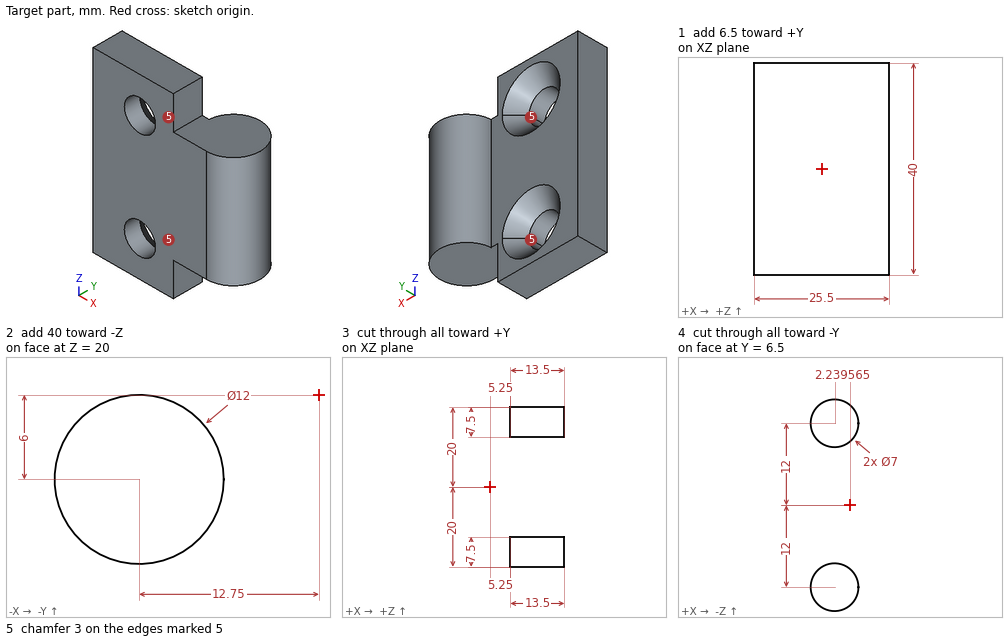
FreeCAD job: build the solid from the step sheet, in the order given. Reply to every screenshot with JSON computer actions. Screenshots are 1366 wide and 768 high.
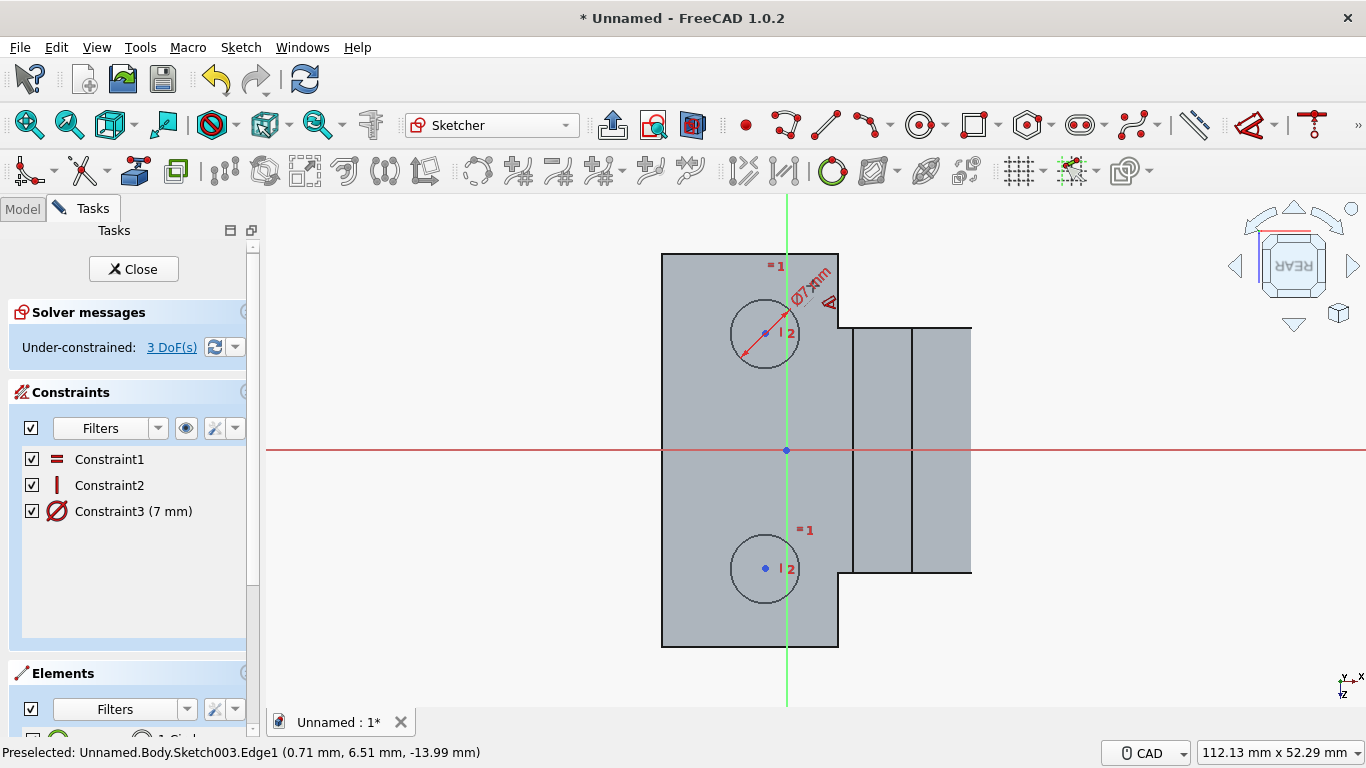
{"action": "left_click", "coordinate": [765, 334]}
{"action": "left_click", "coordinate": [821, 392]}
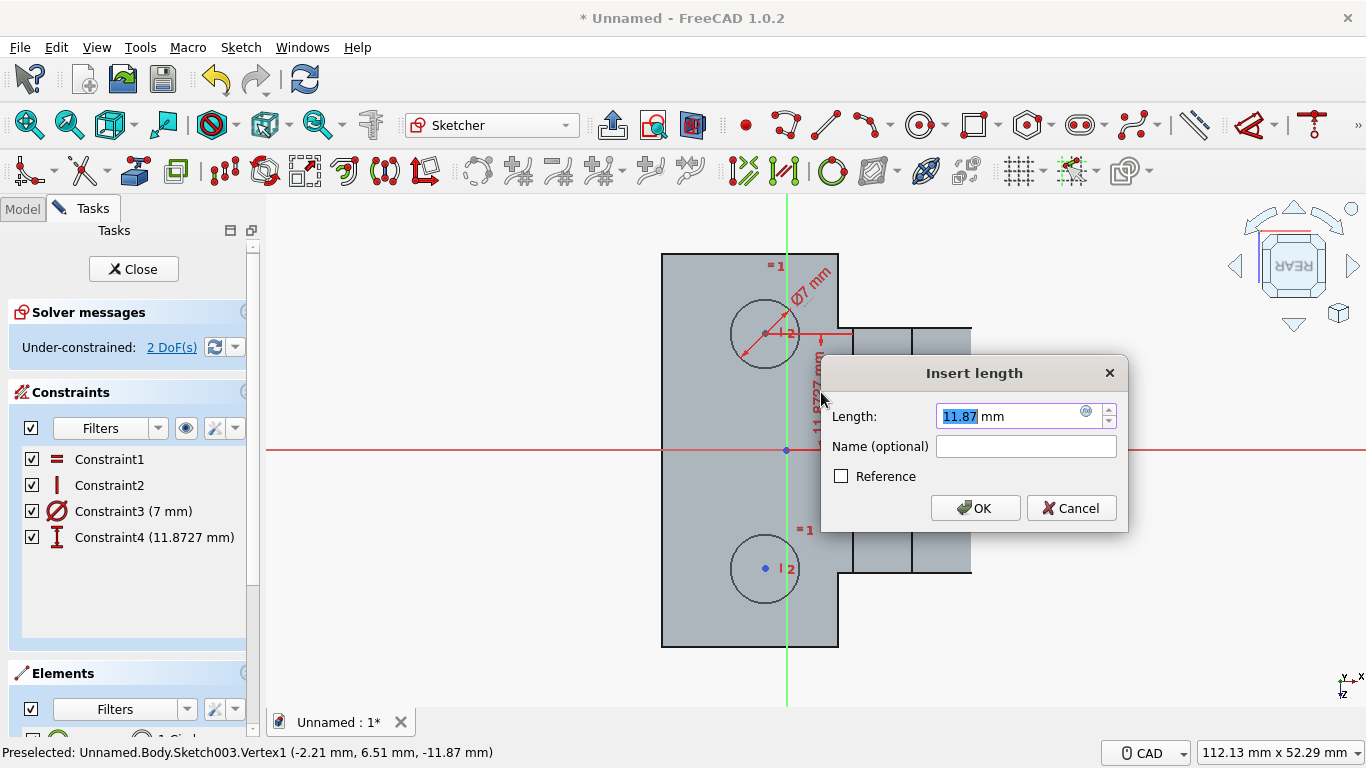
{"action": "type", "text": "12"}
{"action": "key", "text": "Return"}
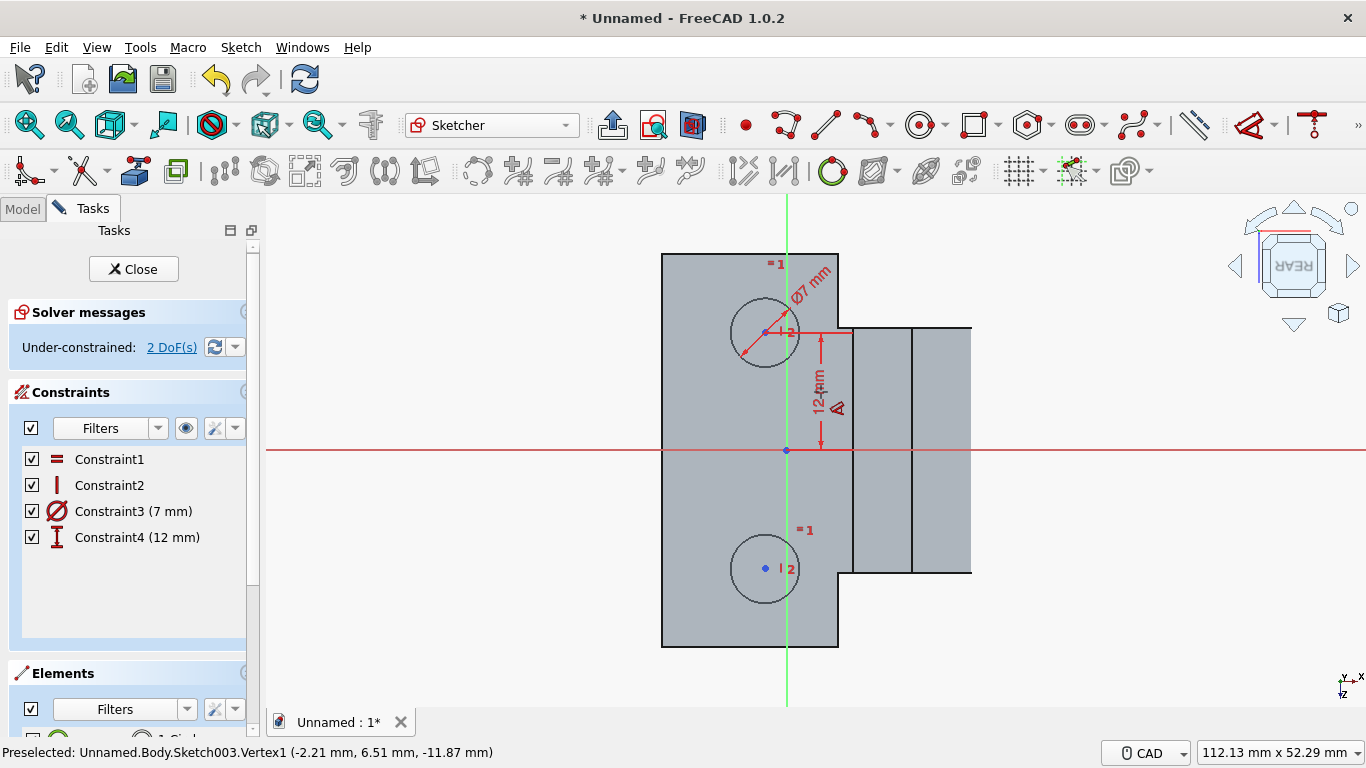
{"action": "left_click", "coordinate": [765, 569]}
{"action": "left_click", "coordinate": [821, 510]}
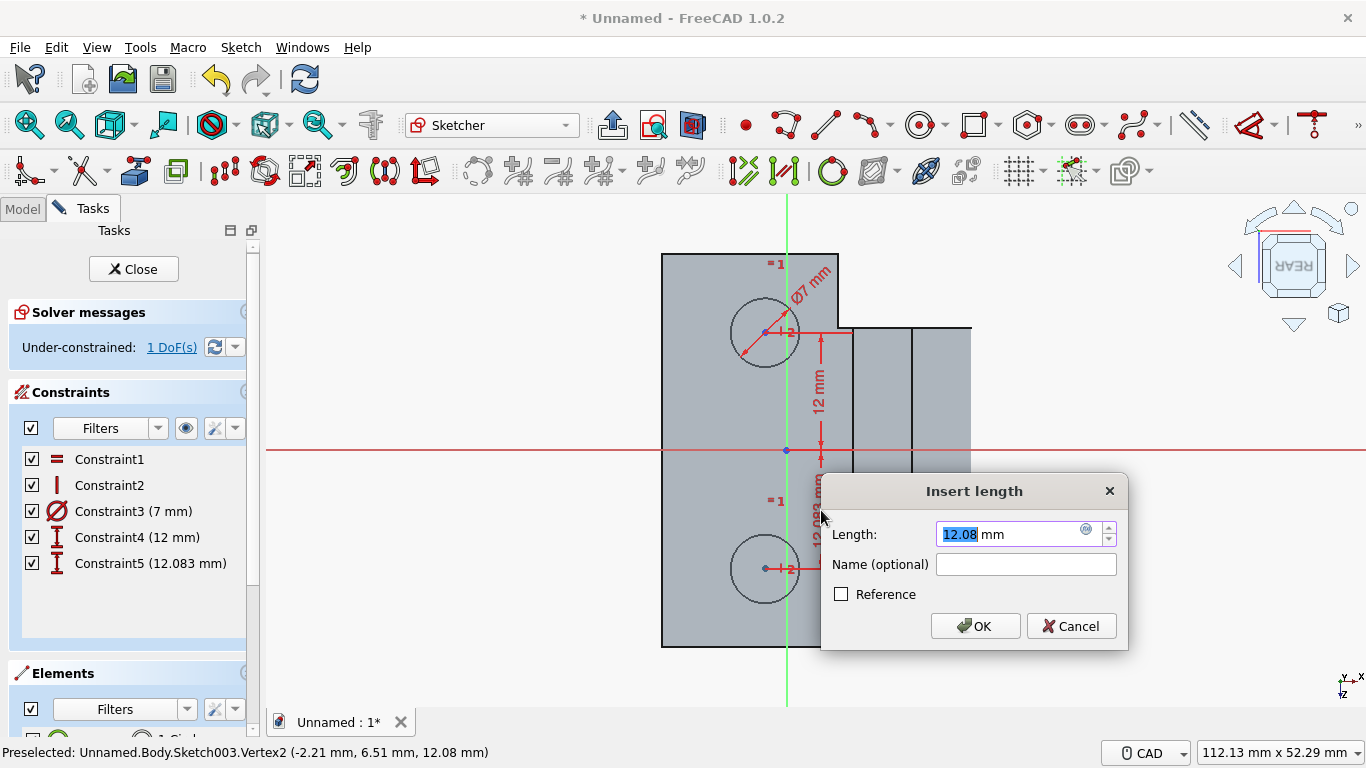
{"action": "type", "text": "12"}
{"action": "key", "text": "Return"}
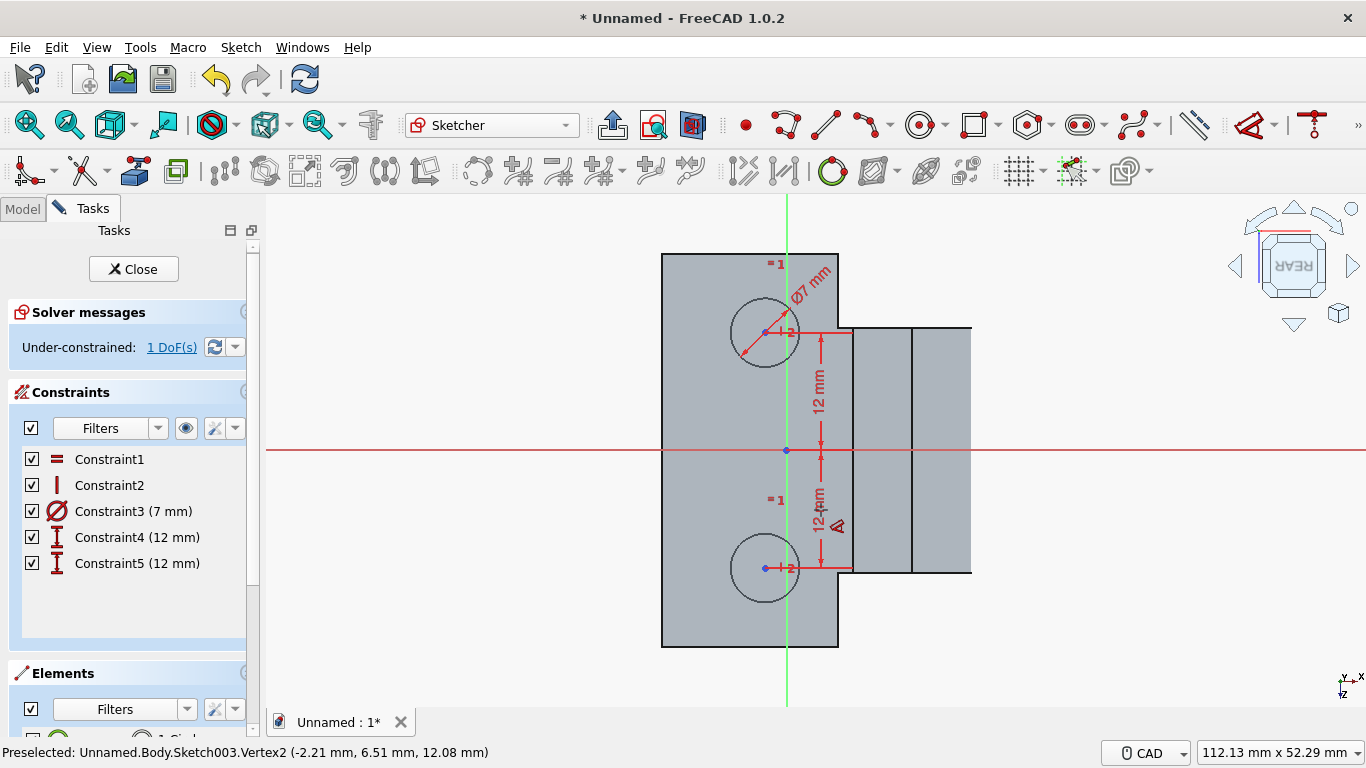
{"action": "scroll", "coordinate": [765, 333], "scroll_direction": "up", "scroll_amount": 3}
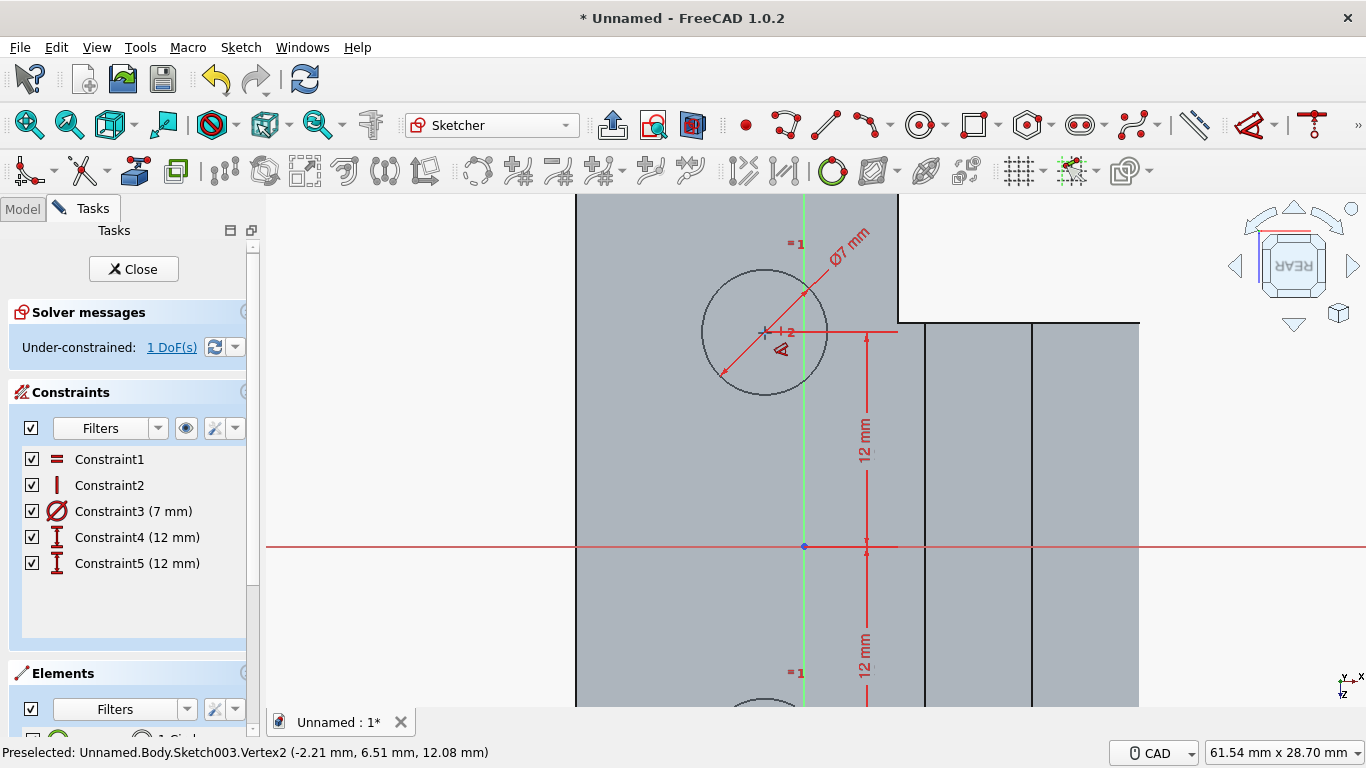
{"action": "left_click", "coordinate": [765, 332]}
{"action": "left_click", "coordinate": [784, 298]}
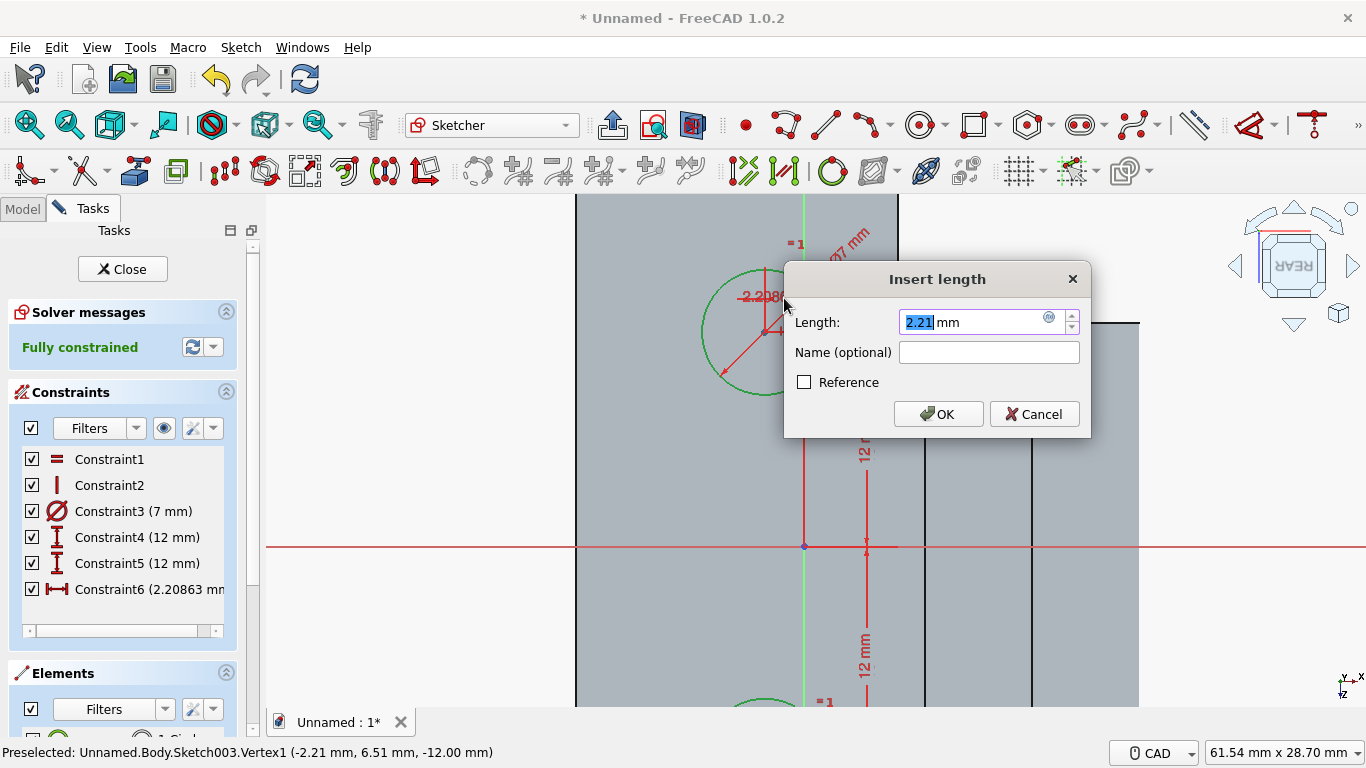
{"action": "type", "text": "2.239565"}
{"action": "key", "text": "Return"}
{"action": "key", "text": "Escape"}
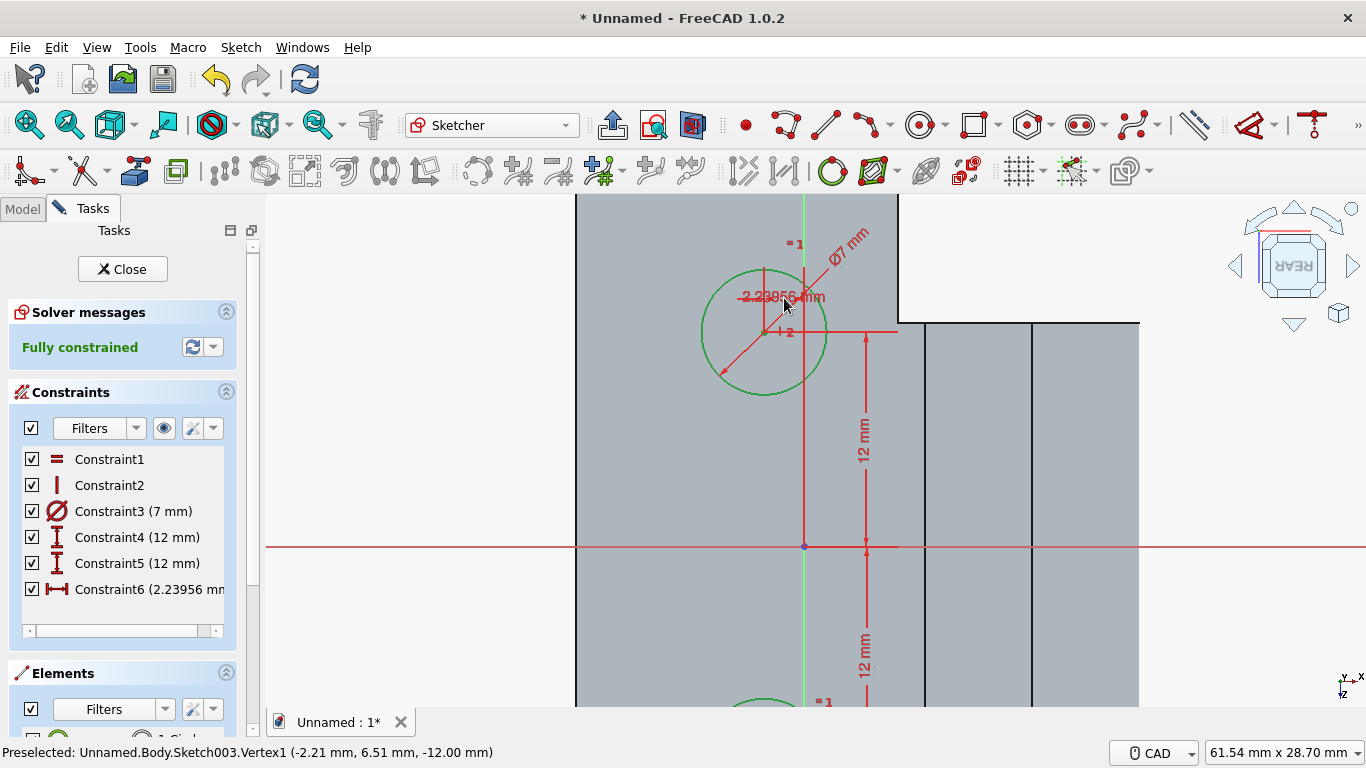
{"action": "left_click", "coordinate": [123, 269]}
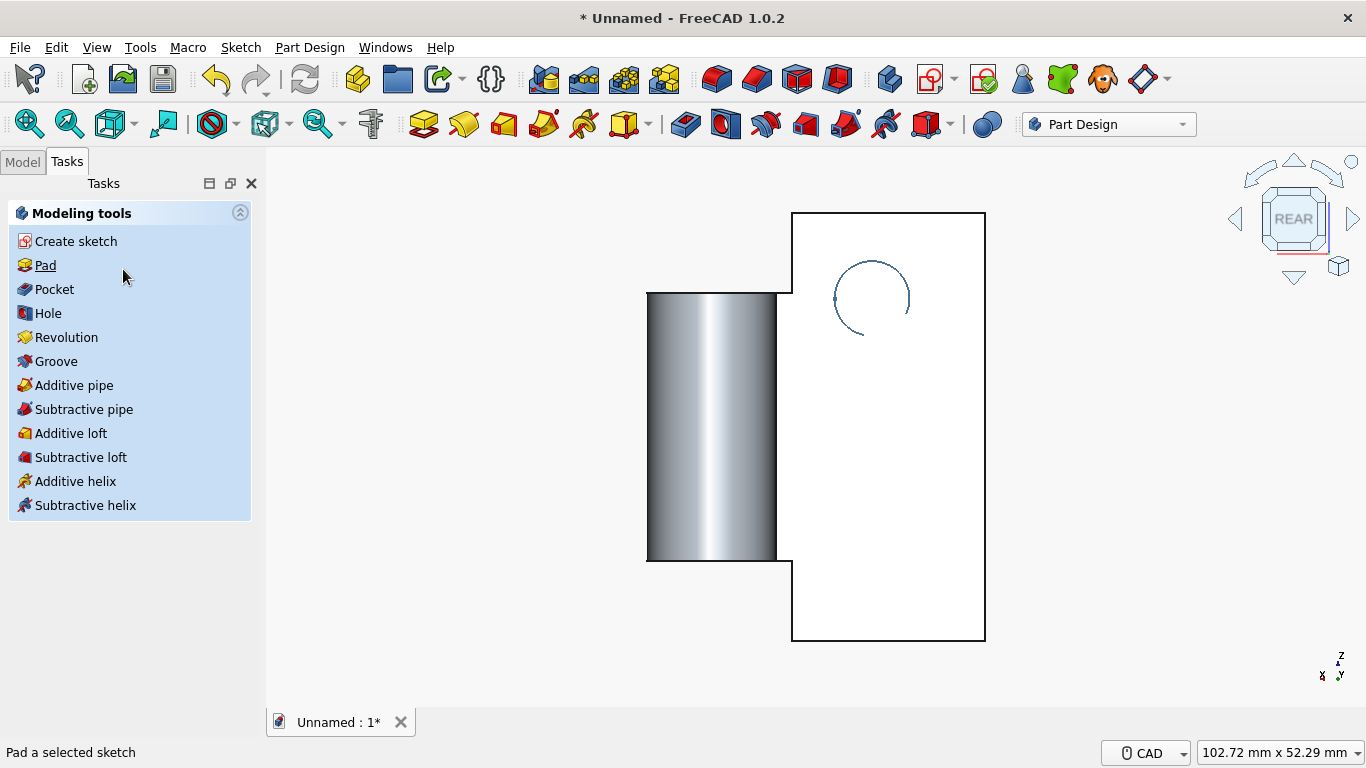
{"action": "left_click", "coordinate": [686, 124]}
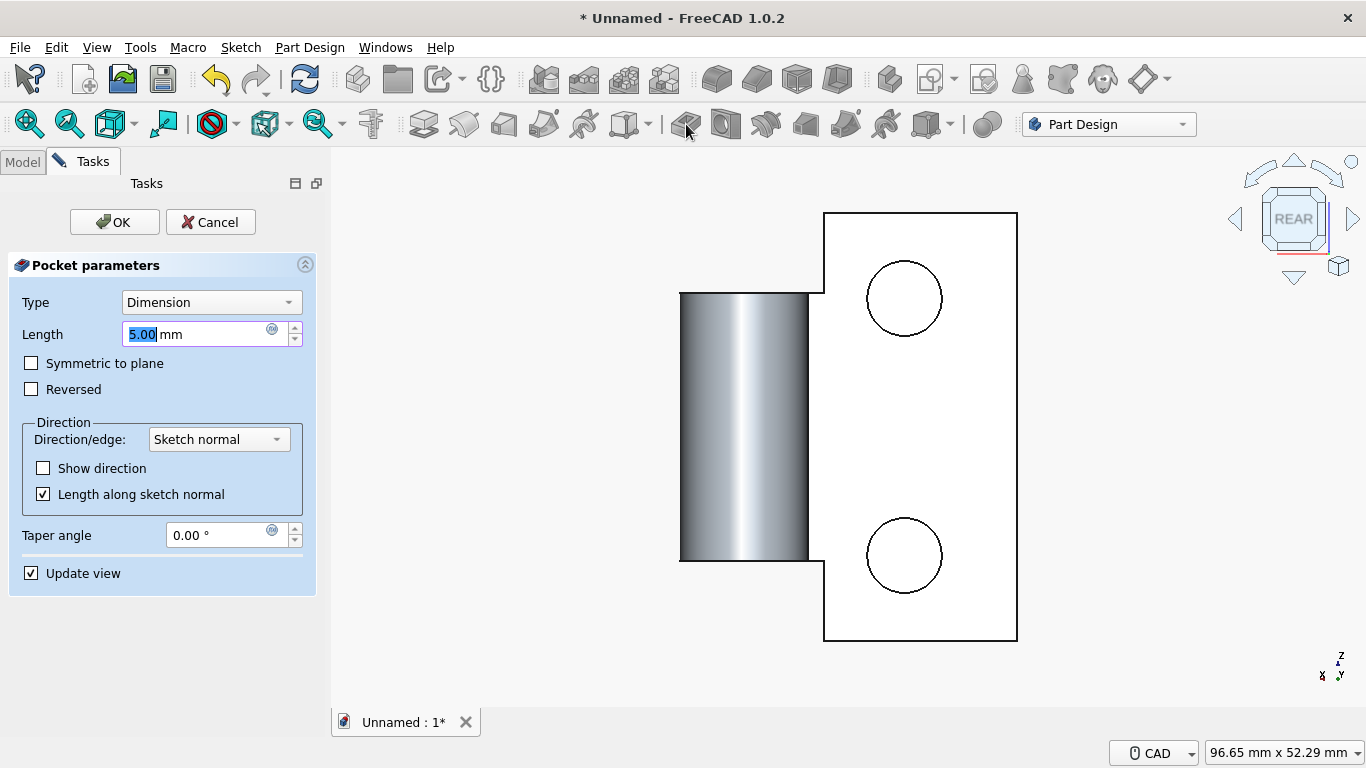
{"action": "left_click", "coordinate": [212, 302]}